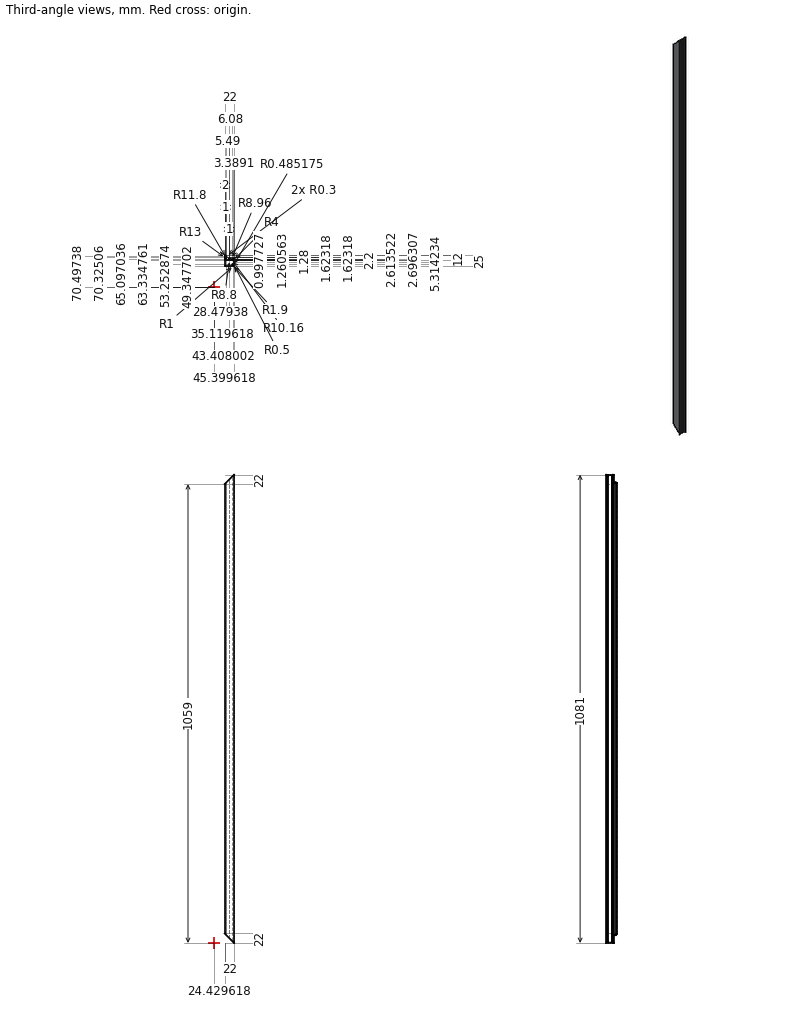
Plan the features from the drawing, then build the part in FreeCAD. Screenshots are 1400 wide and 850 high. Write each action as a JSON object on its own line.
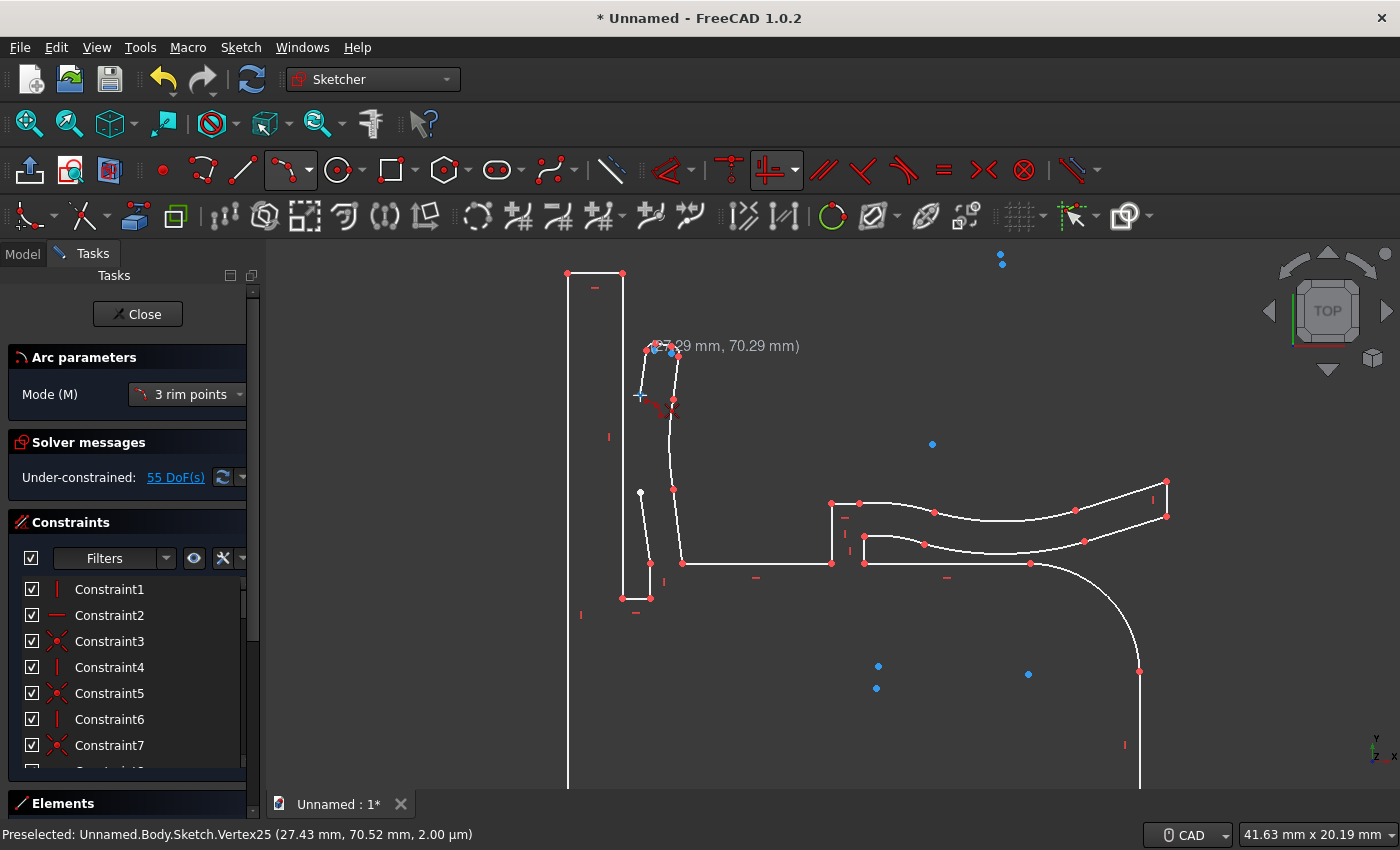
{"action": "left_click", "coordinate": [640, 395]}
{"action": "left_click", "coordinate": [640, 493]}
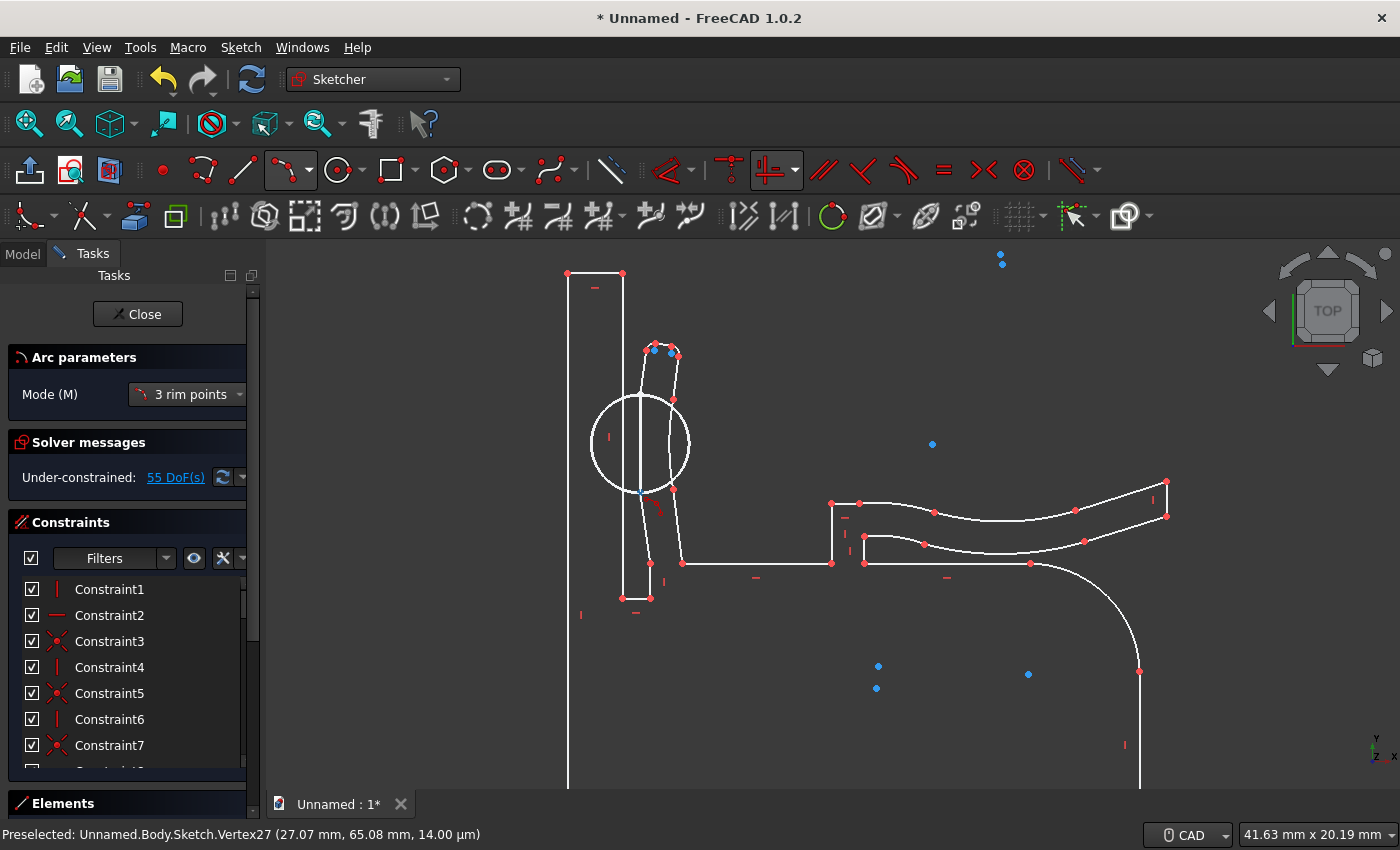
{"action": "scroll", "coordinate": [637, 443], "scroll_direction": "up", "scroll_amount": 8}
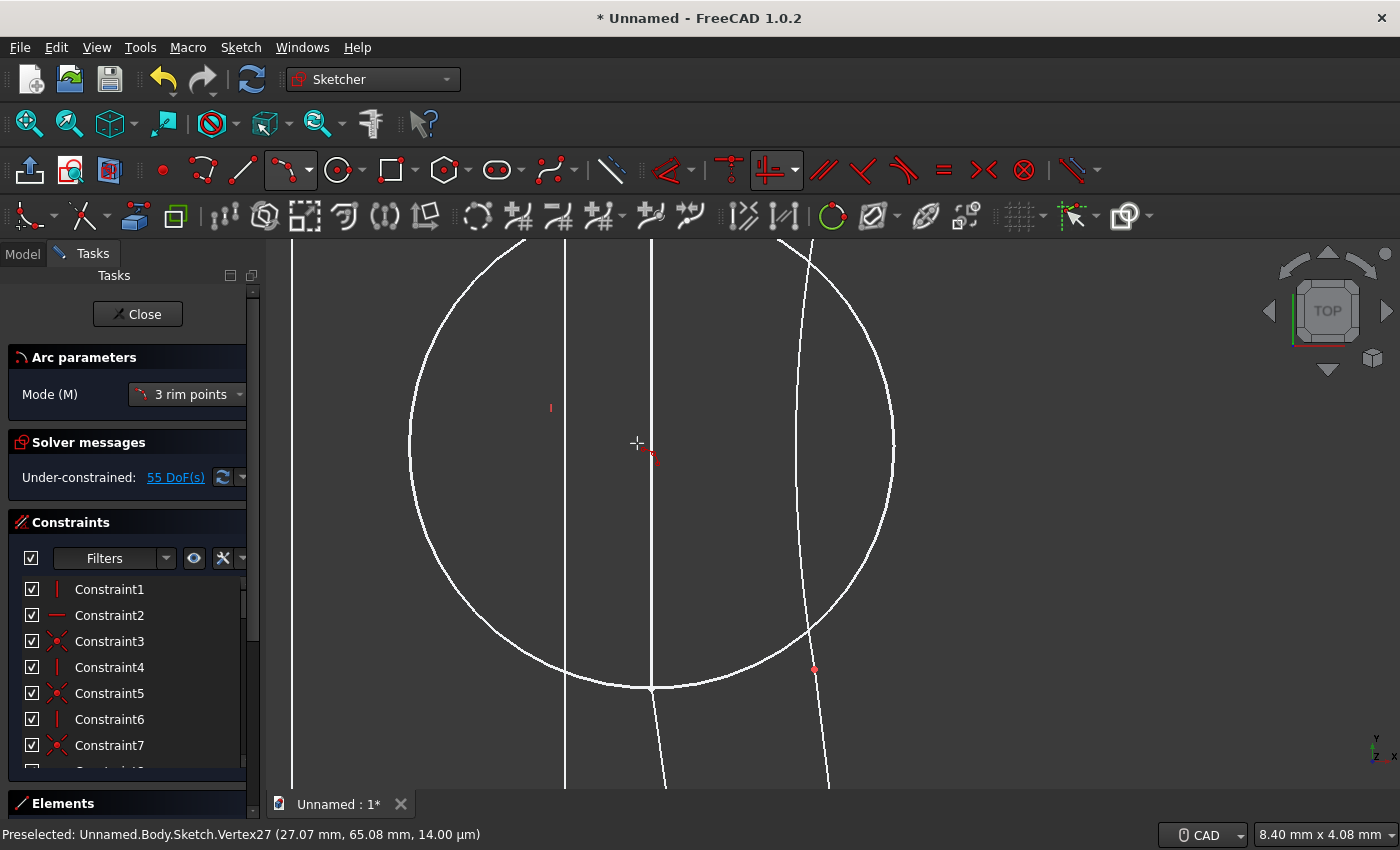
{"action": "left_click", "coordinate": [634, 443]}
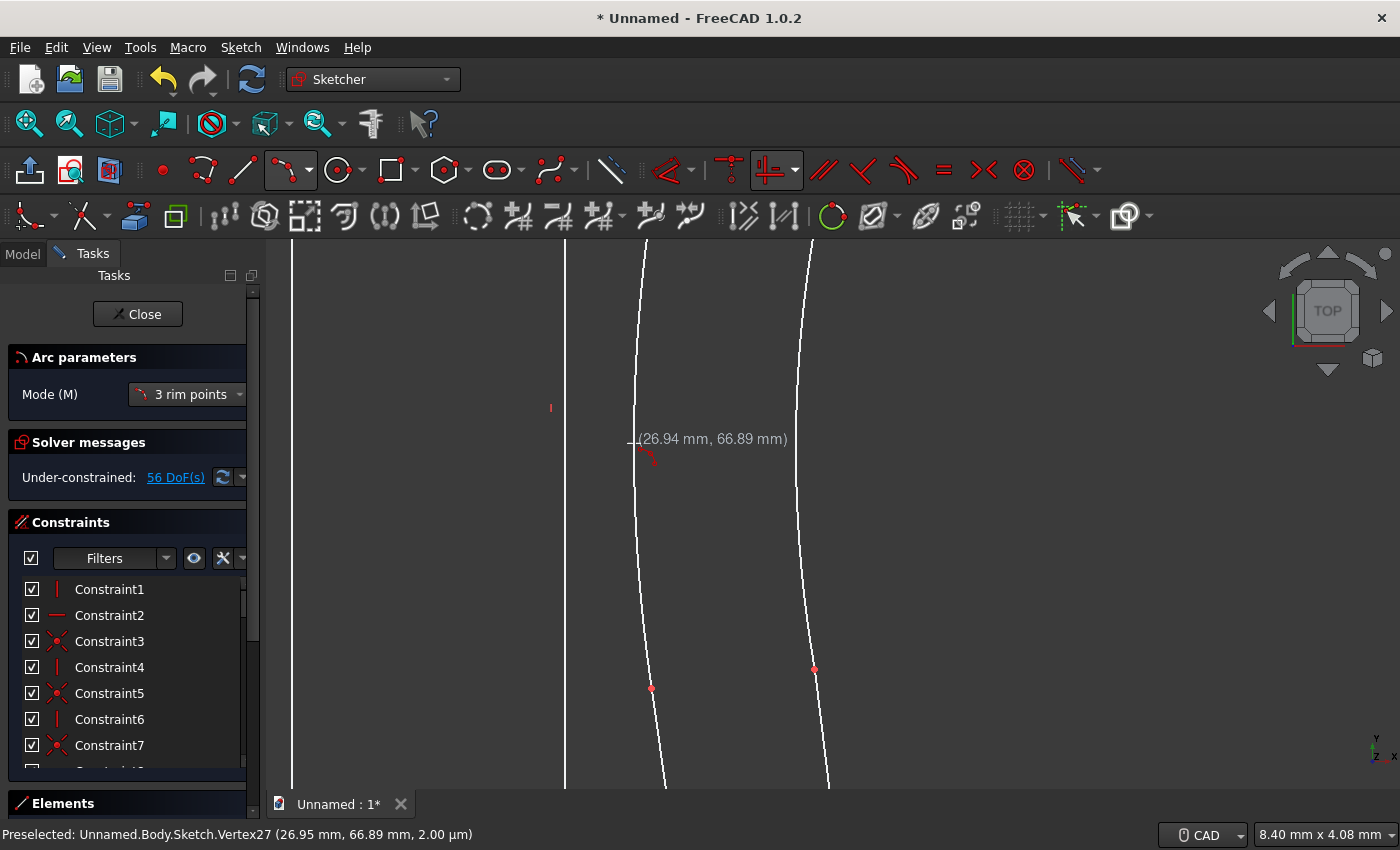
{"action": "scroll", "coordinate": [638, 419], "scroll_direction": "down", "scroll_amount": 11}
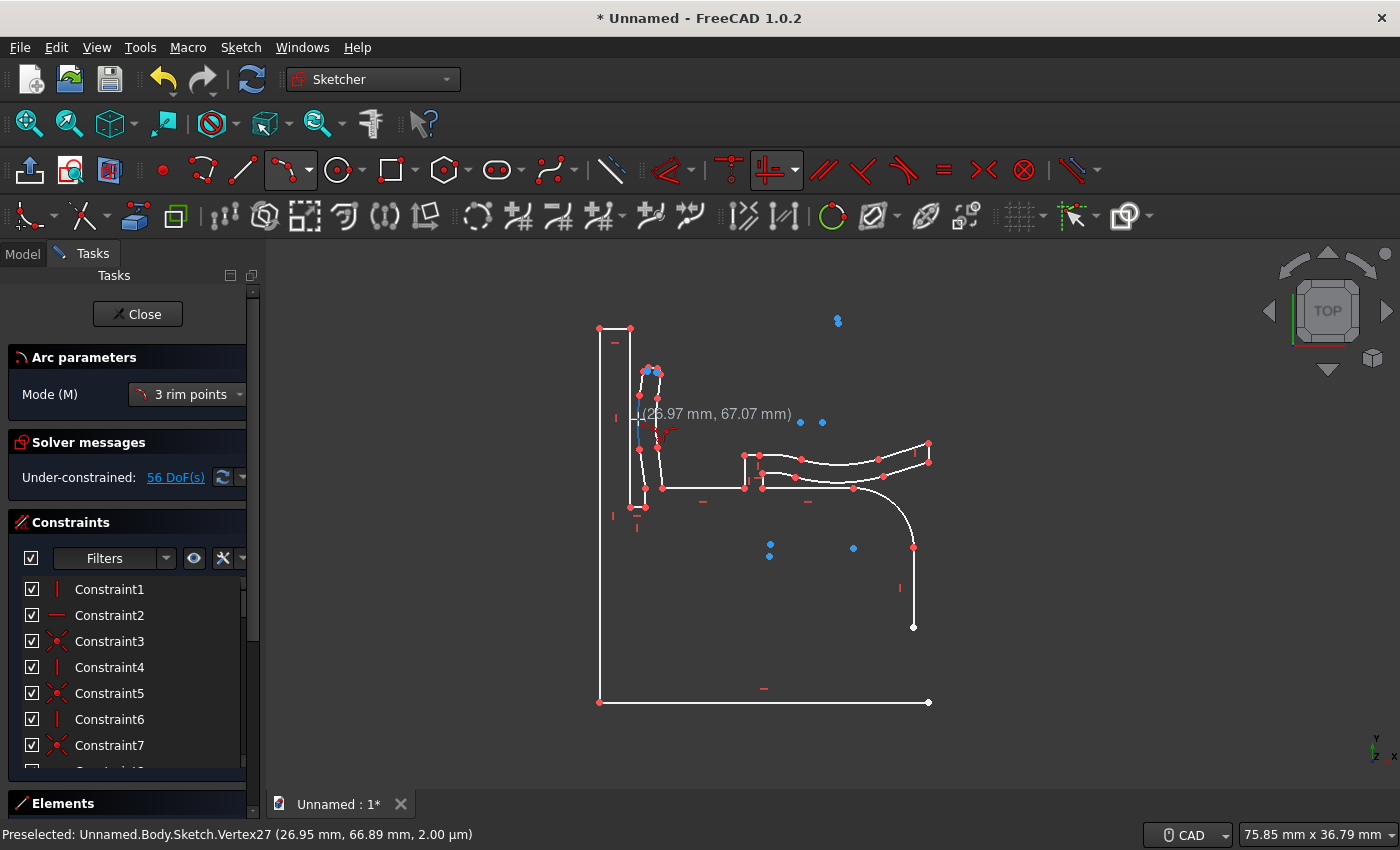
{"action": "left_click", "coordinate": [929, 703]}
{"action": "left_click", "coordinate": [914, 684]}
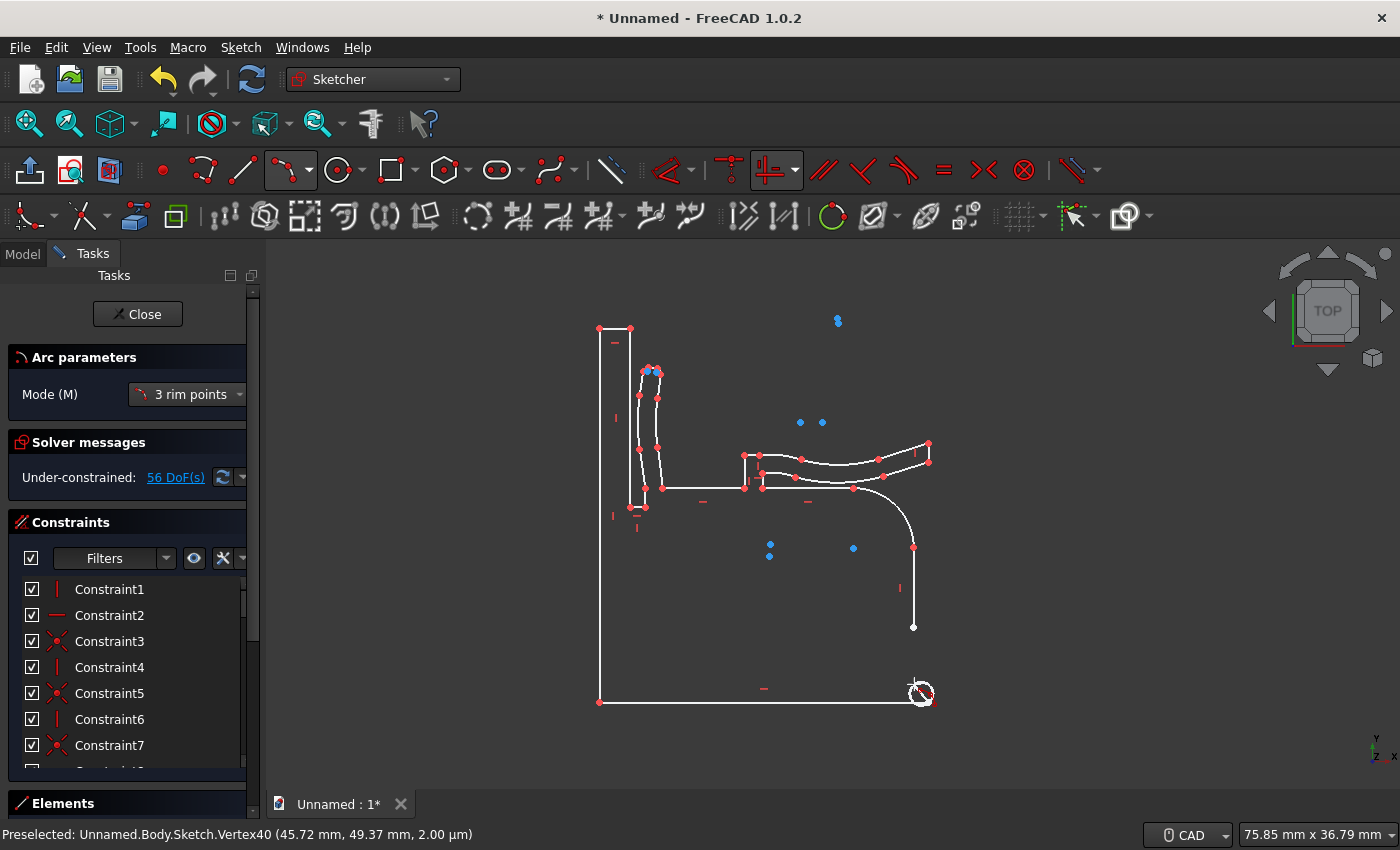
{"action": "scroll", "coordinate": [918, 696], "scroll_direction": "up", "scroll_amount": 6}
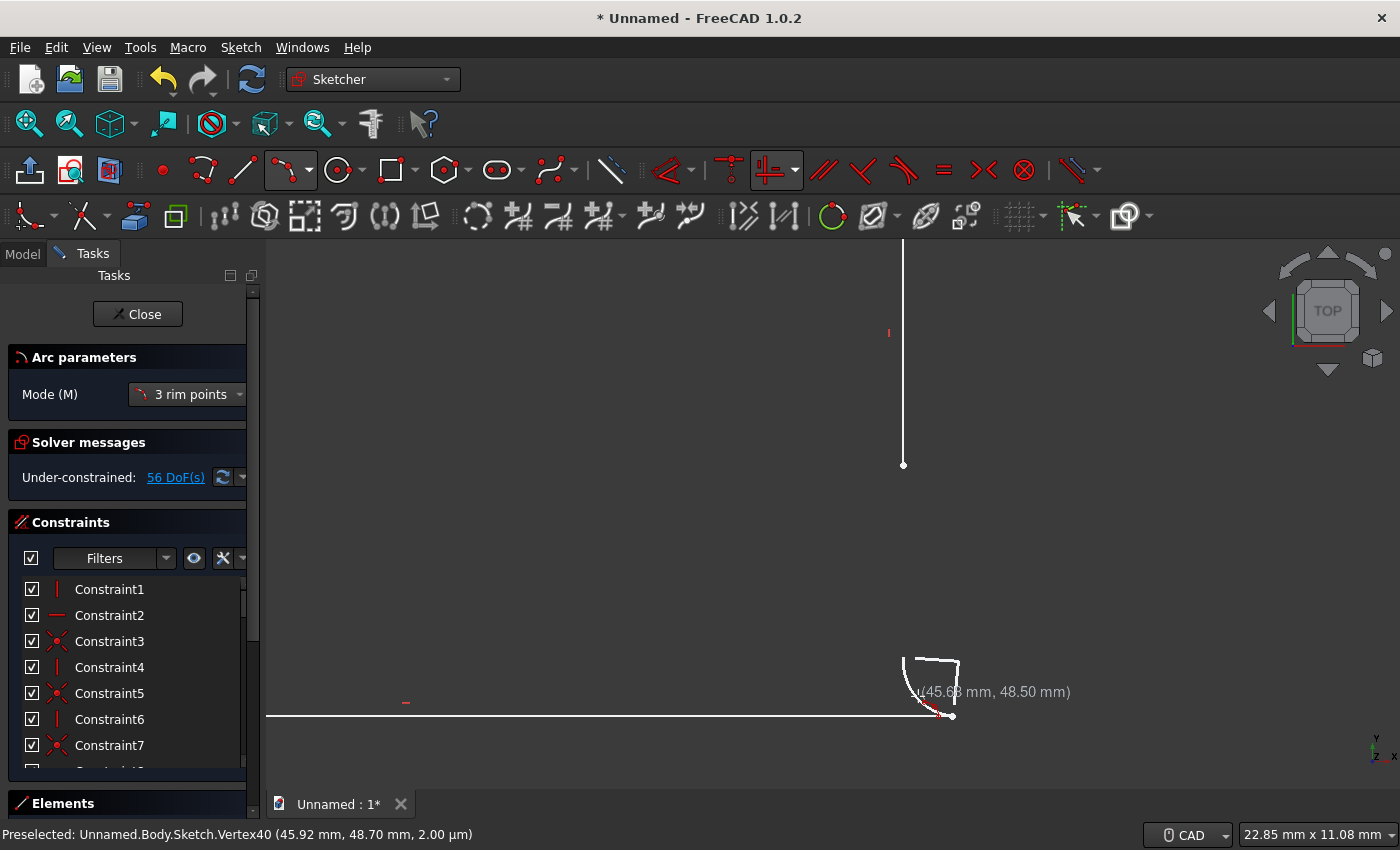
{"action": "left_click", "coordinate": [916, 695]}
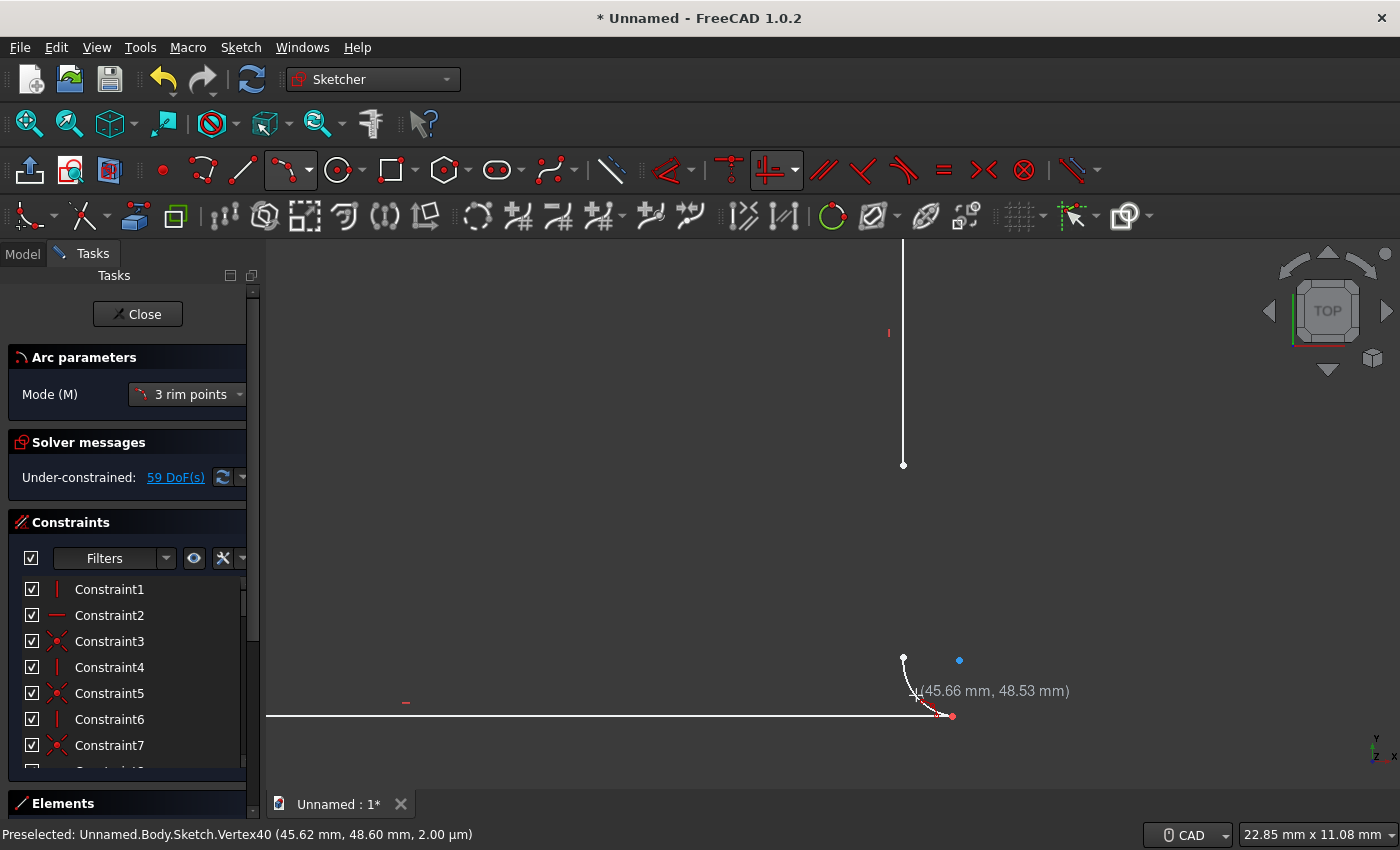
{"action": "left_click", "coordinate": [903, 658]}
{"action": "left_click", "coordinate": [866, 633]}
{"action": "left_click", "coordinate": [893, 631]}